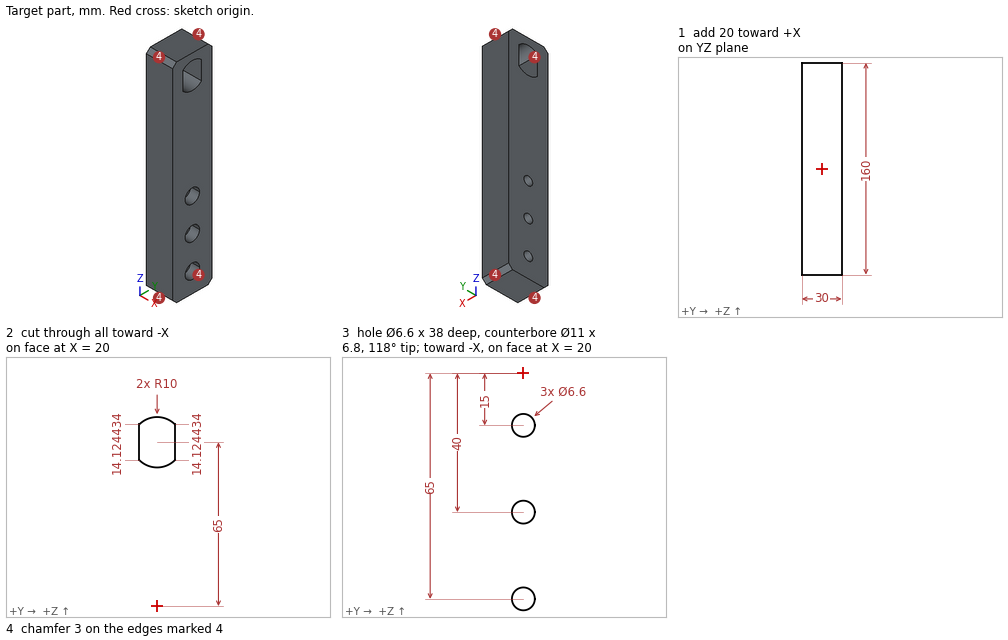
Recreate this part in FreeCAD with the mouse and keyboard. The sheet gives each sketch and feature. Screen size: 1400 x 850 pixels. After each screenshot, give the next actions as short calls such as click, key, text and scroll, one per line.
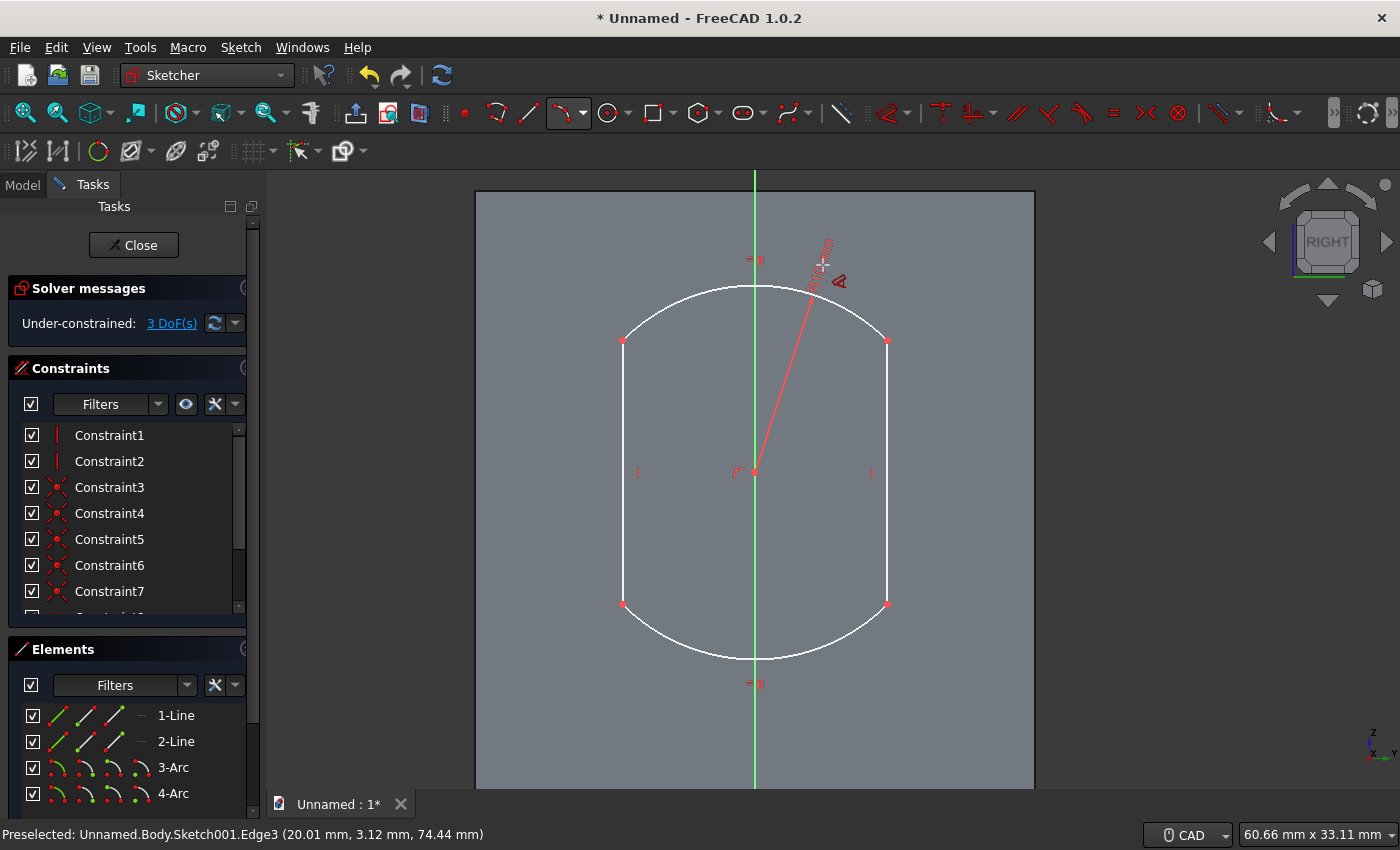
click(755, 473)
click(789, 617)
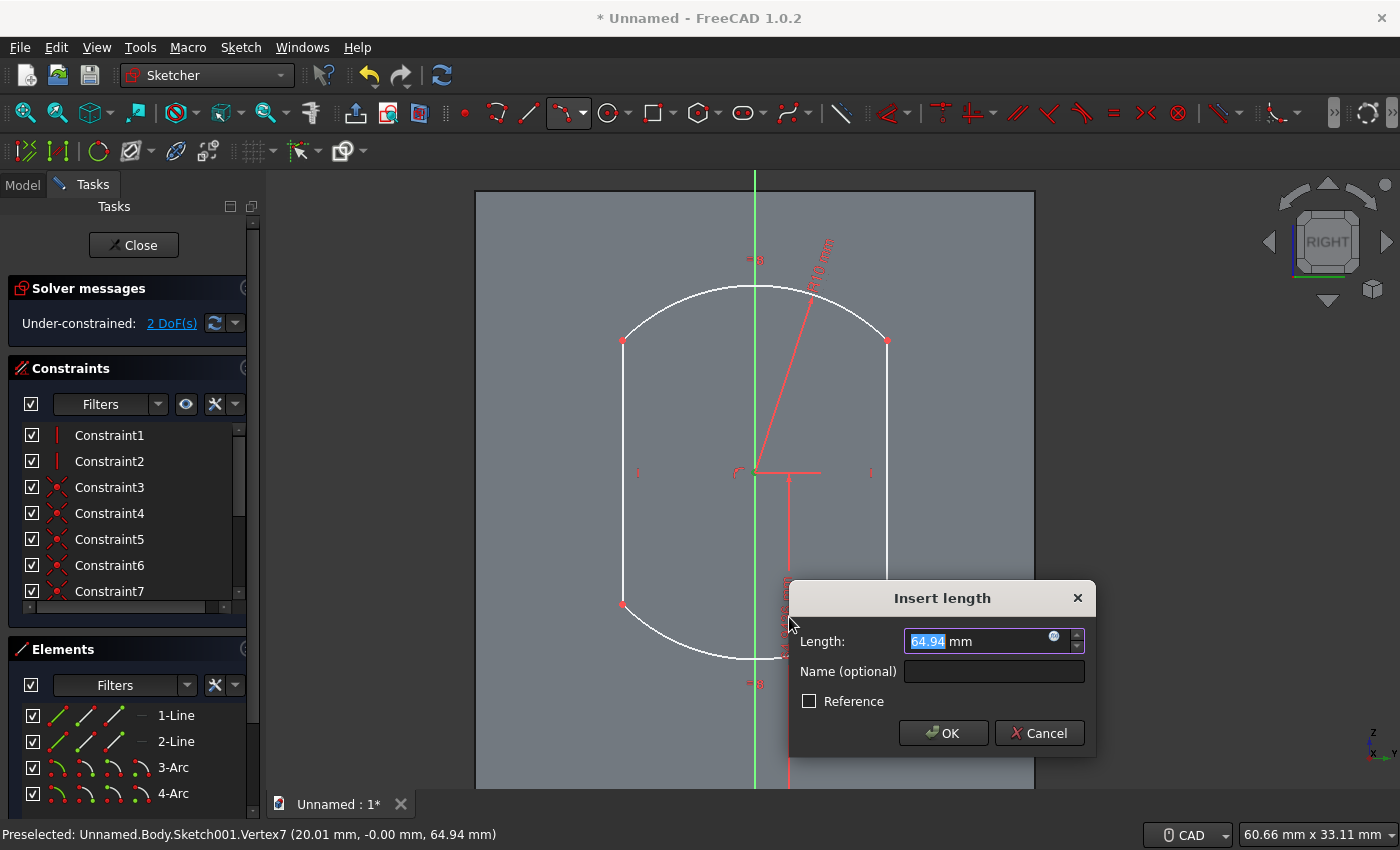
text(65)
key(Return)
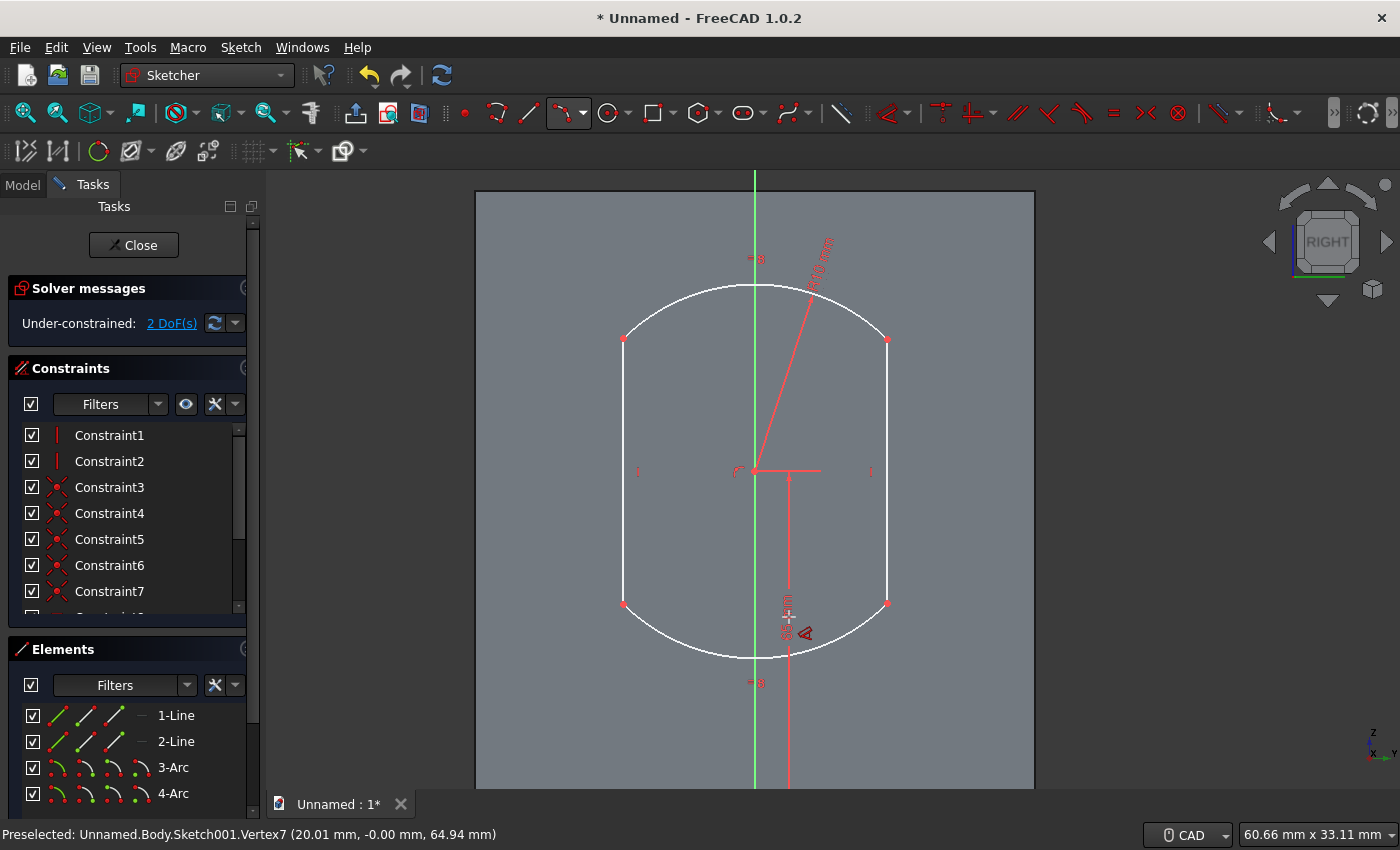
click(887, 524)
click(921, 471)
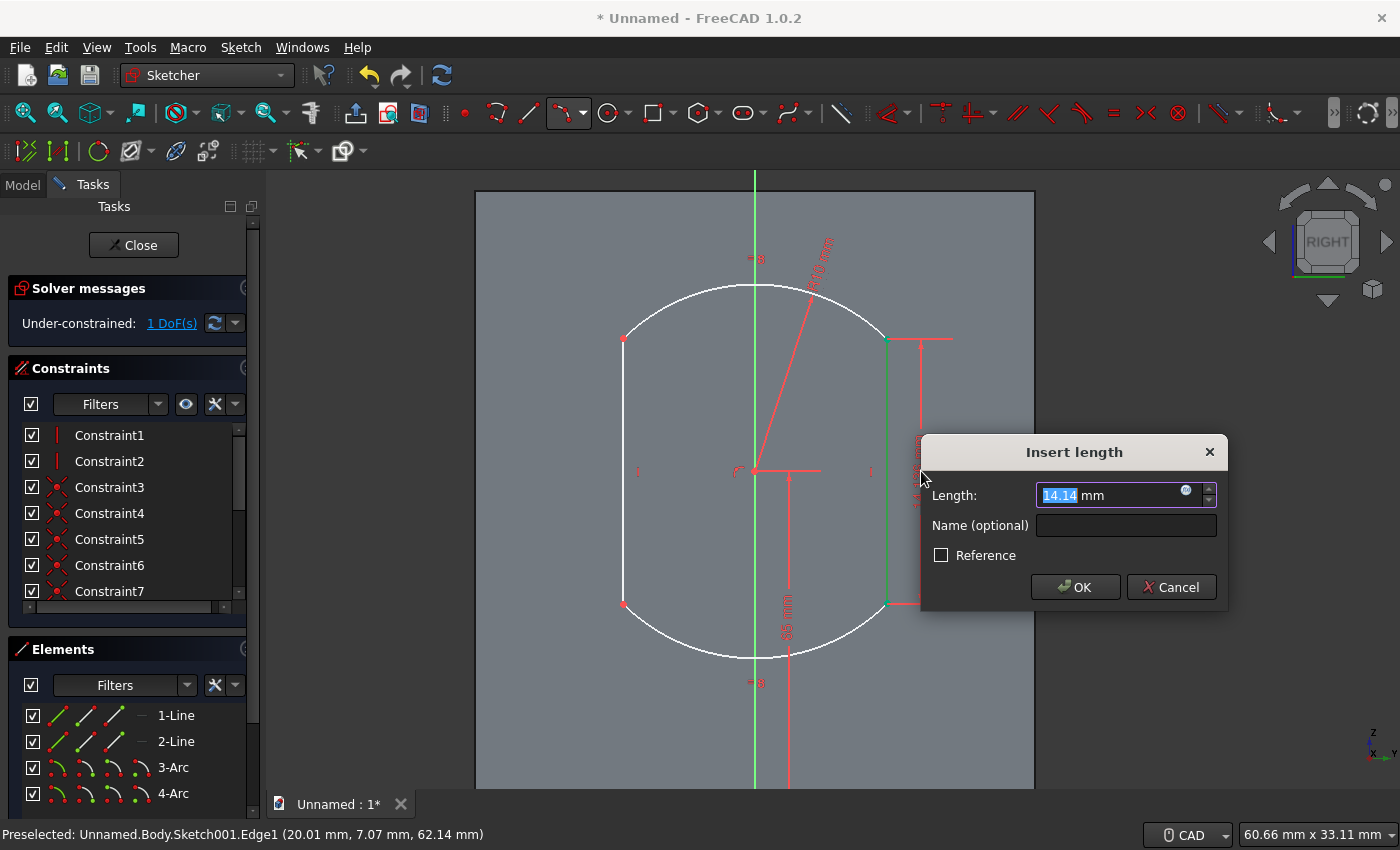
text(14.124434)
key(Return)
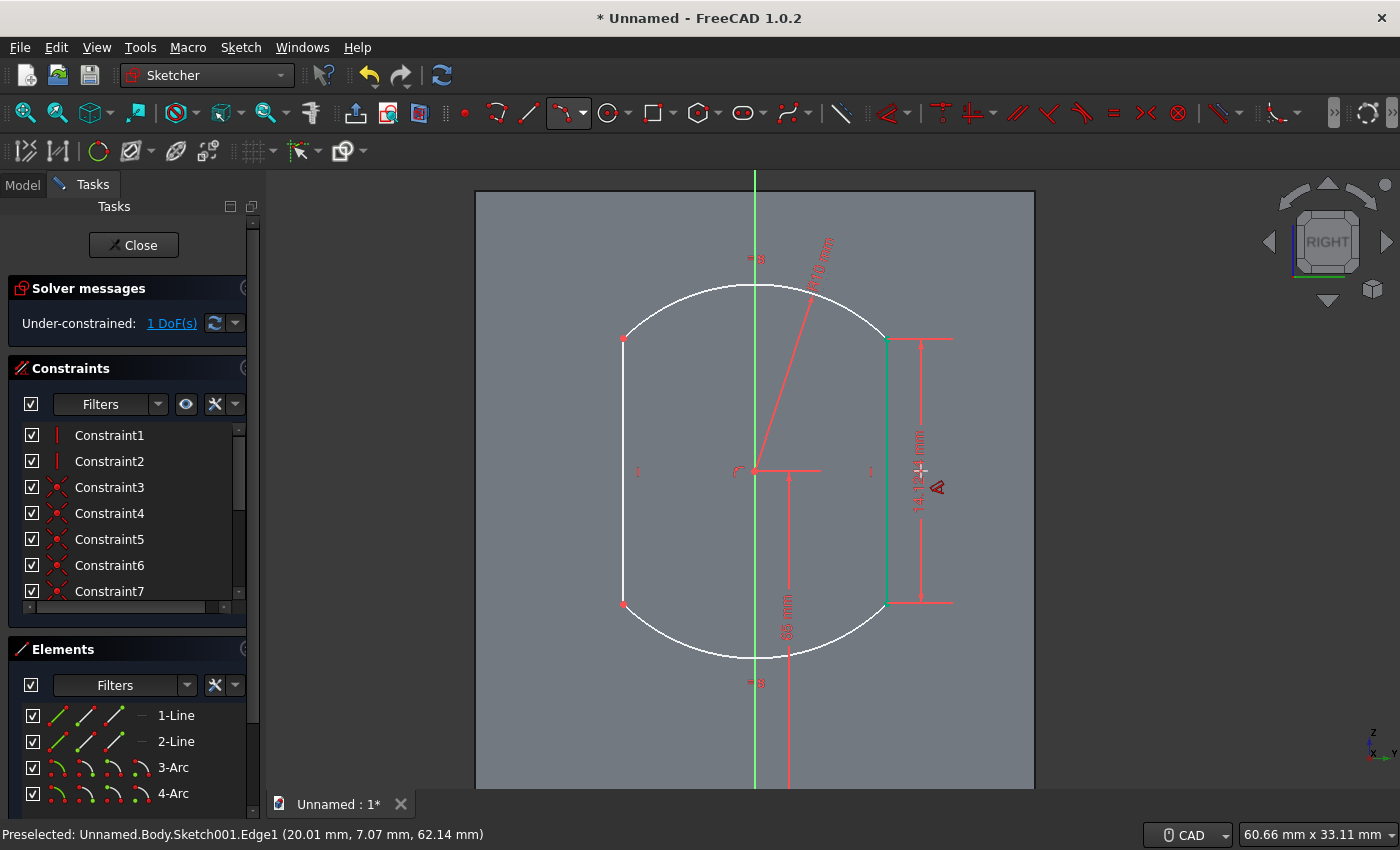
click(623, 418)
click(589, 471)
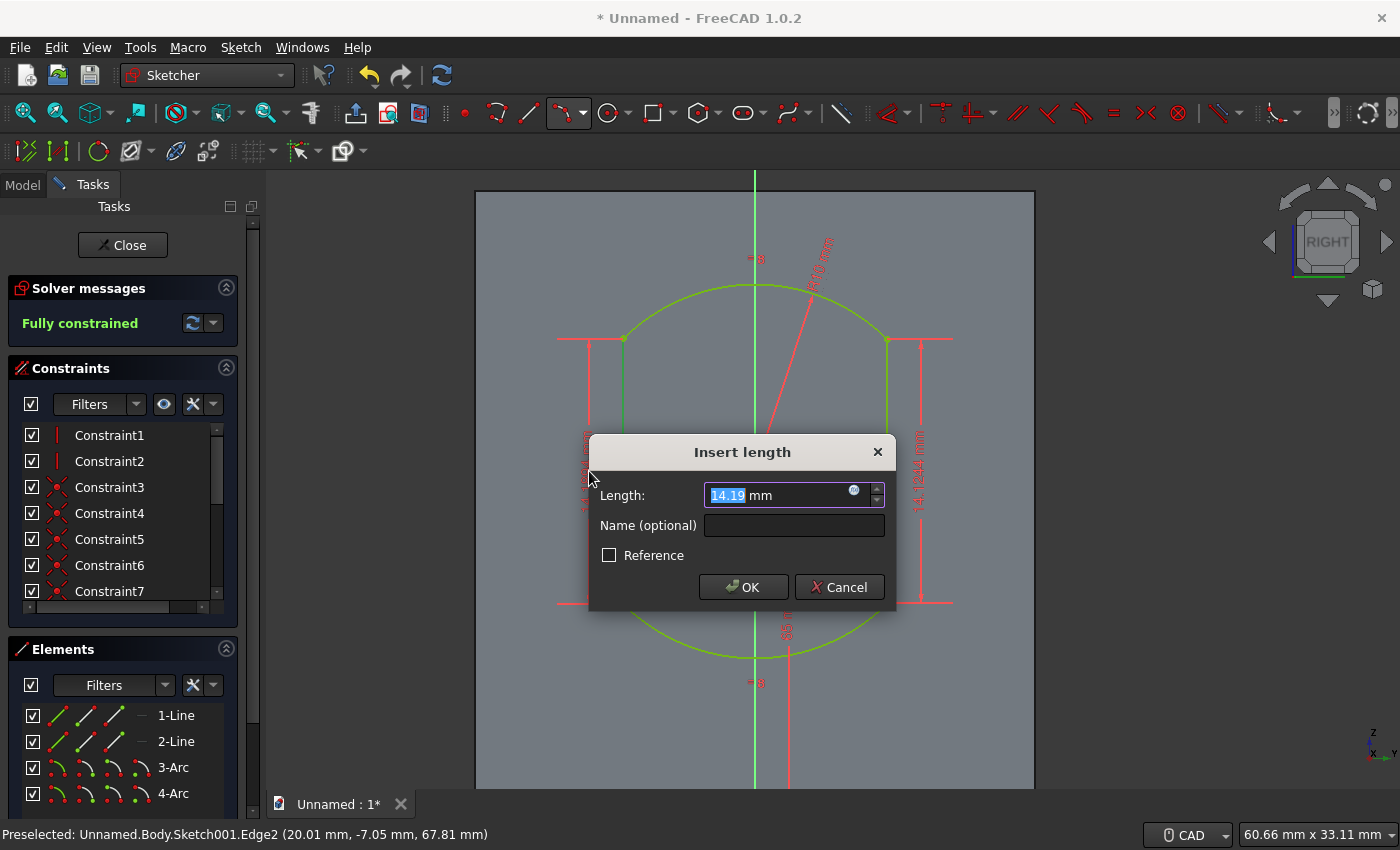
text(14.124434)
key(Return)
key(Escape)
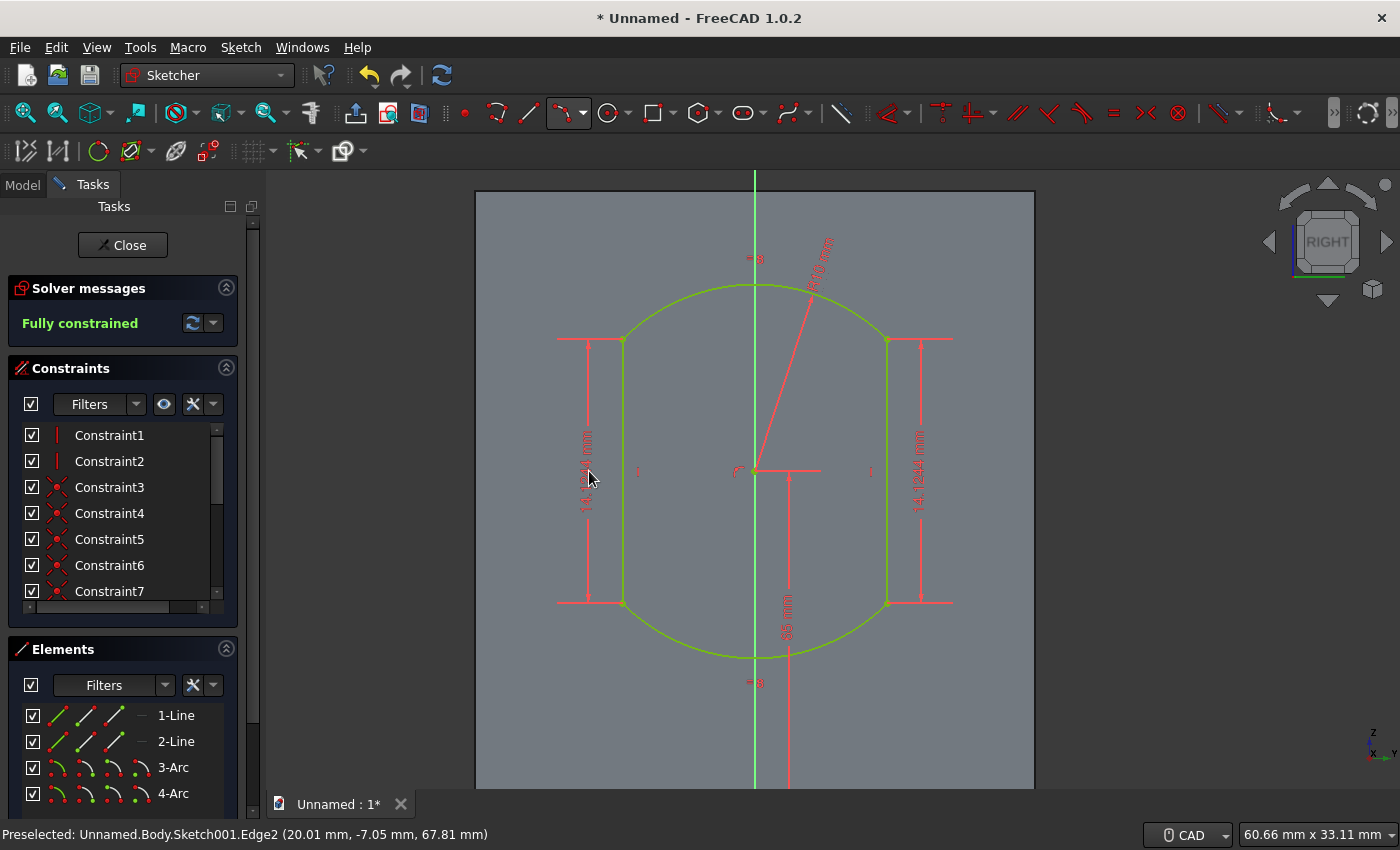
click(123, 245)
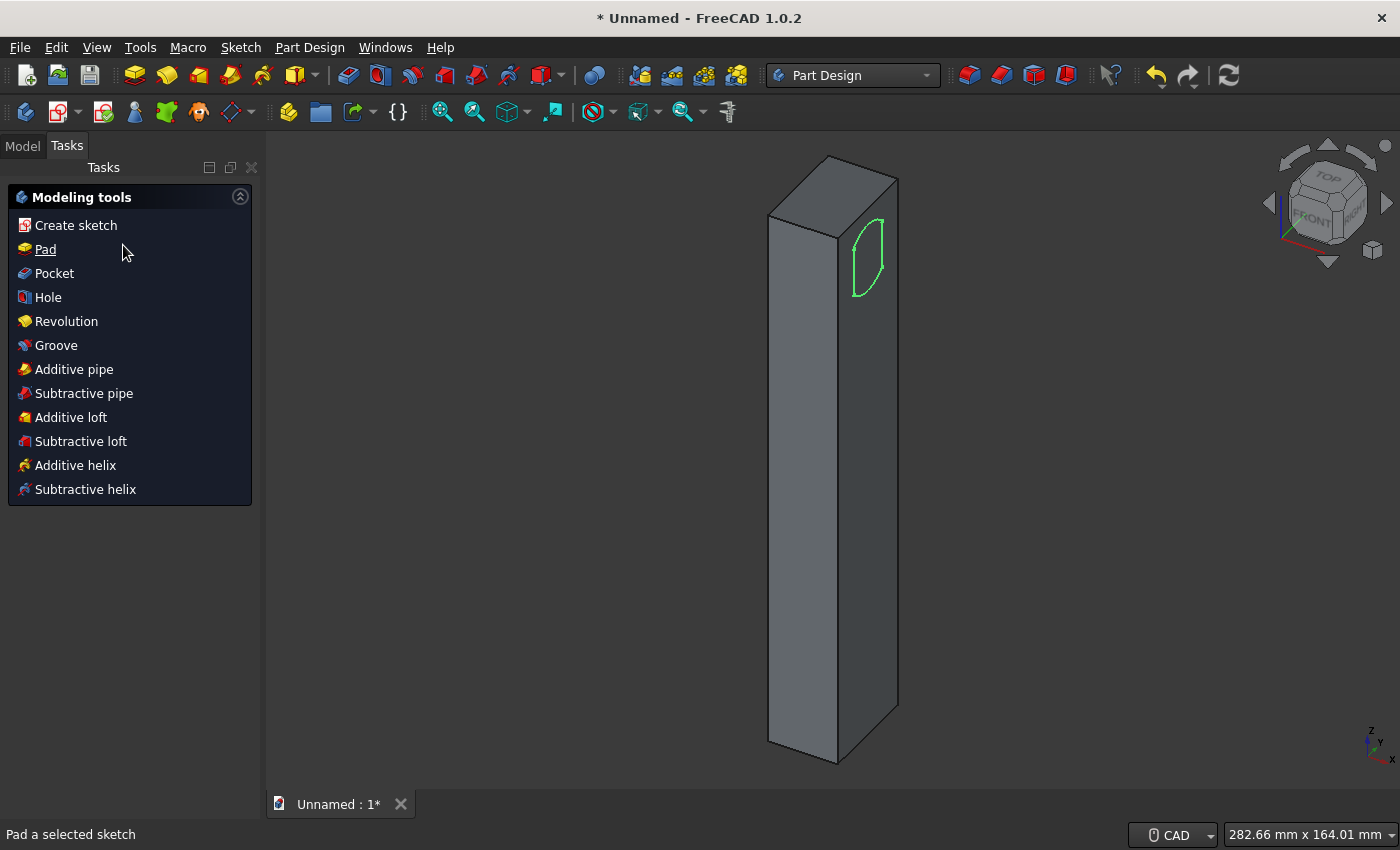
click(350, 76)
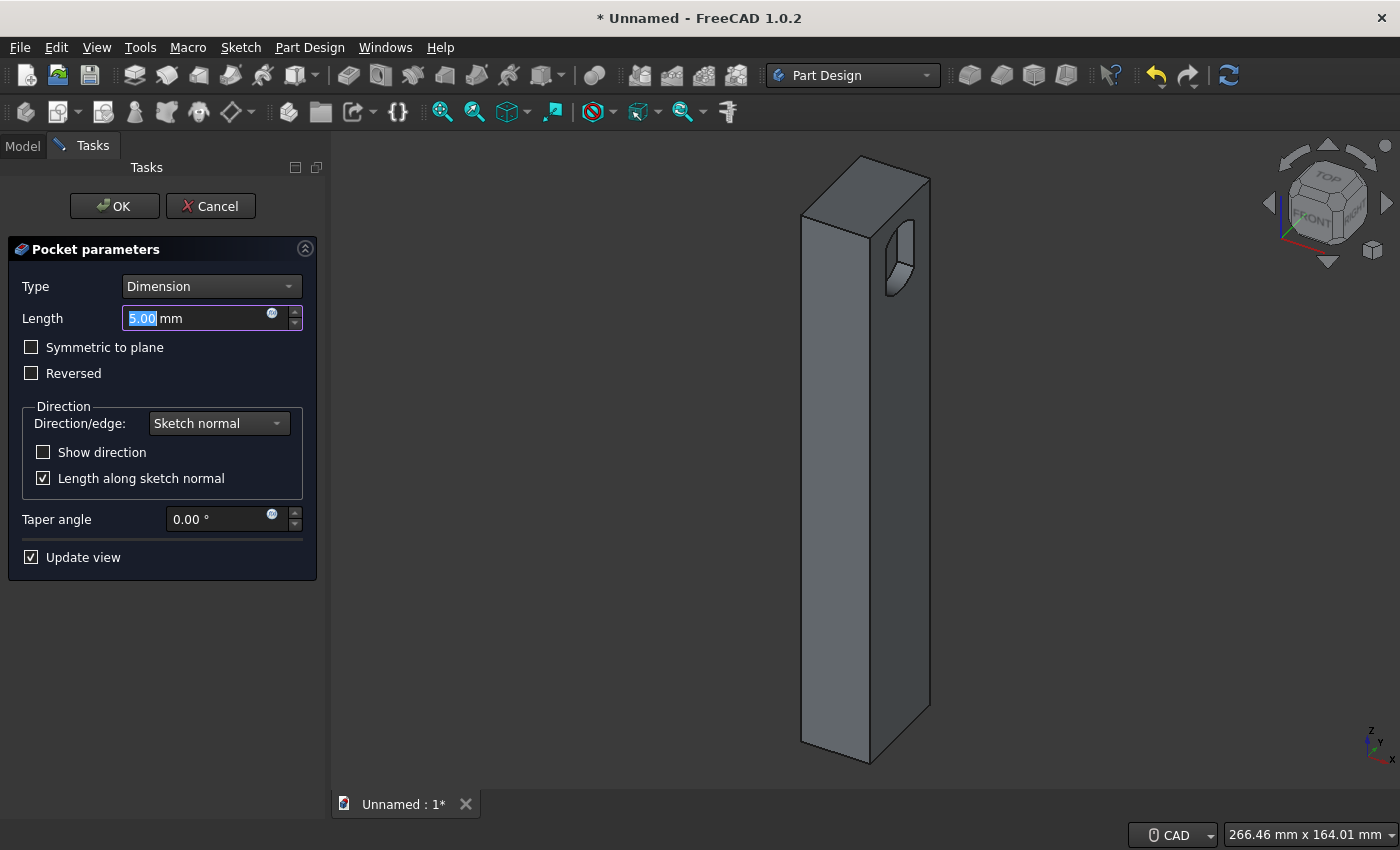
click(212, 286)